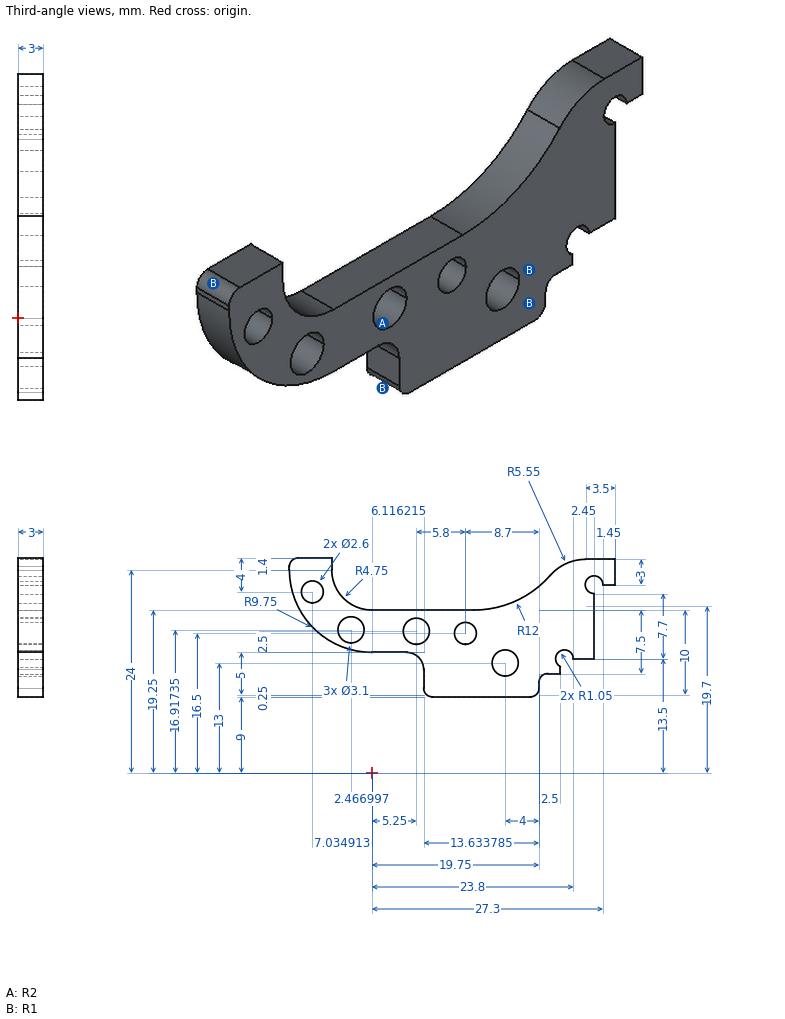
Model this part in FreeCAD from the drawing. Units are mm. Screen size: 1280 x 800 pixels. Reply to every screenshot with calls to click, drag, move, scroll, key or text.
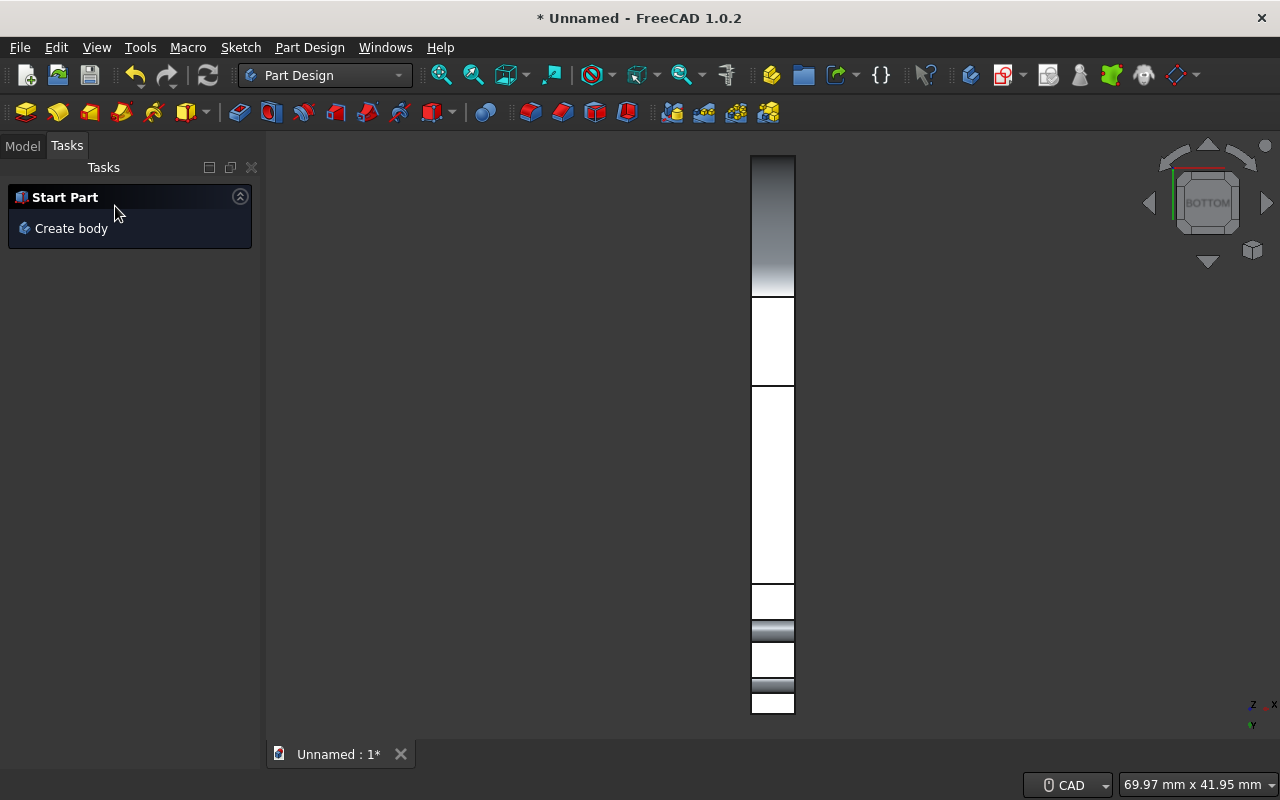
key(4)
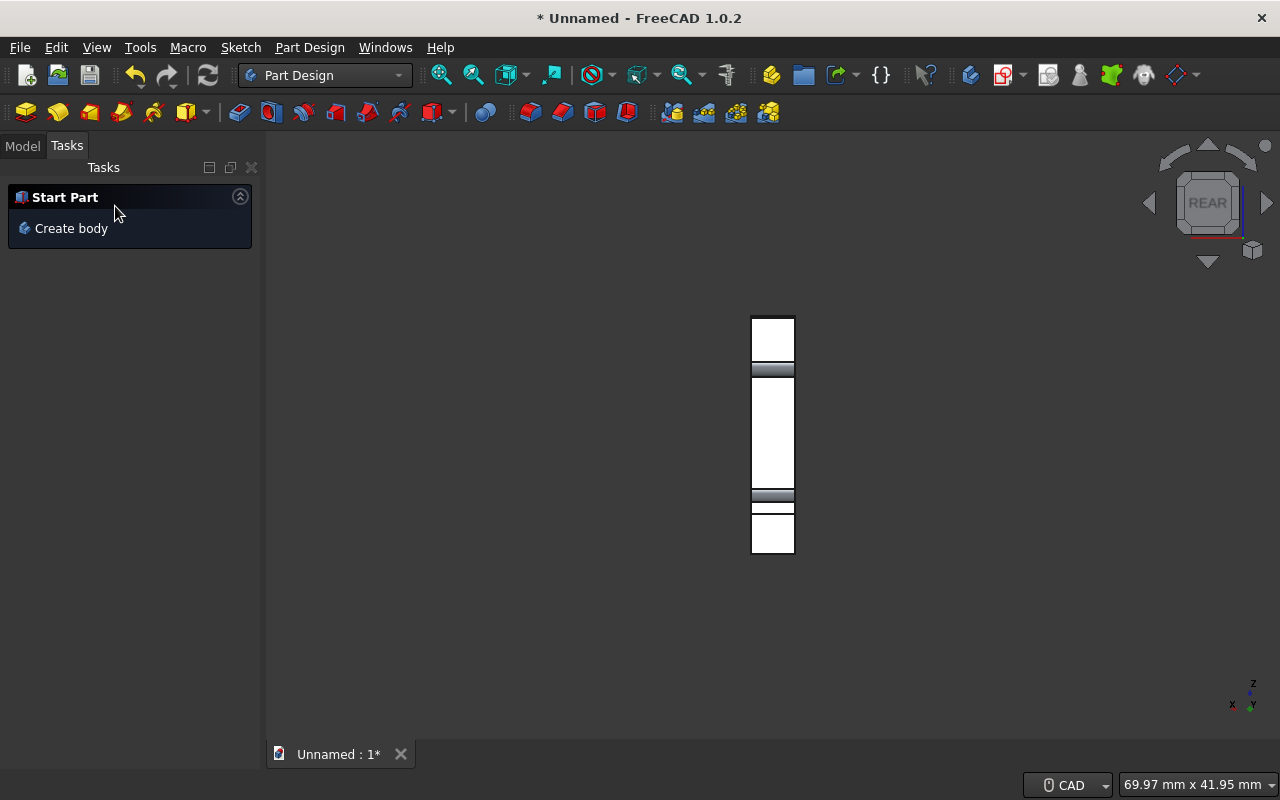
key(v)
key(f)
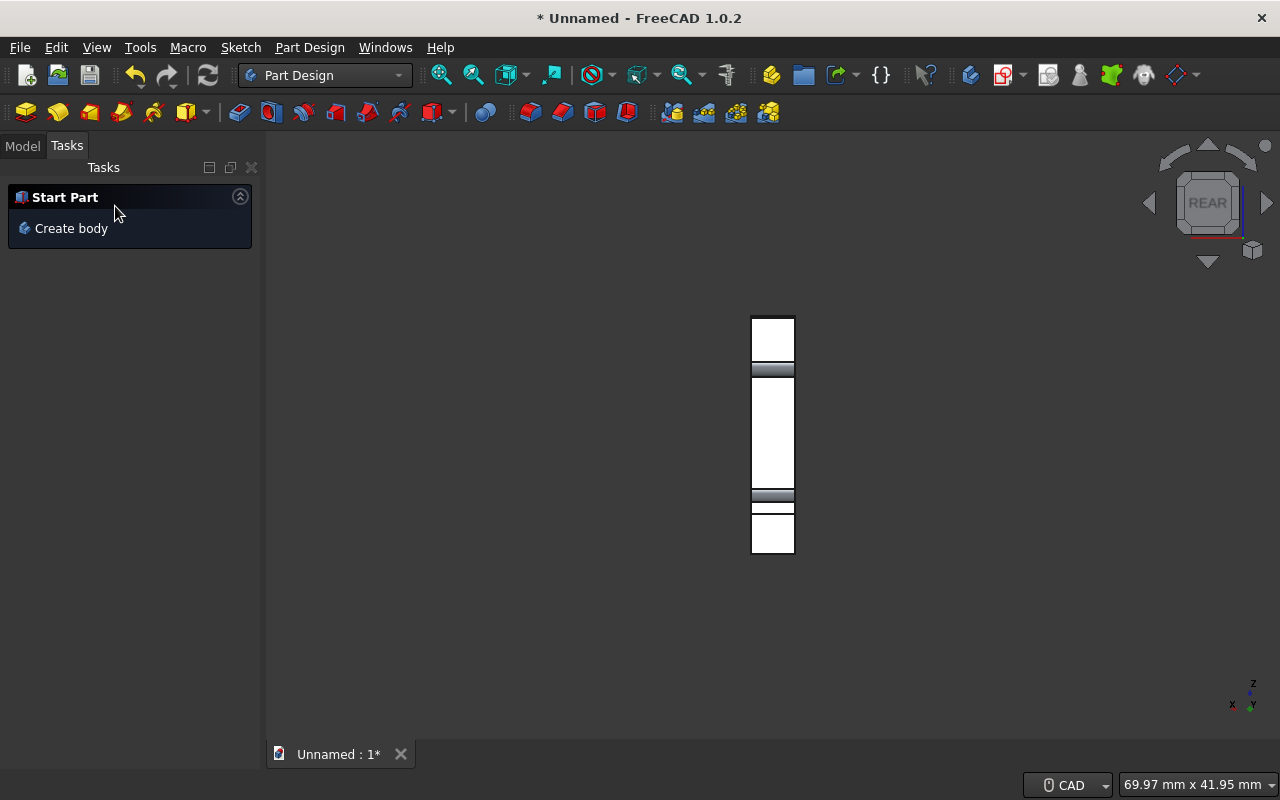
key(6)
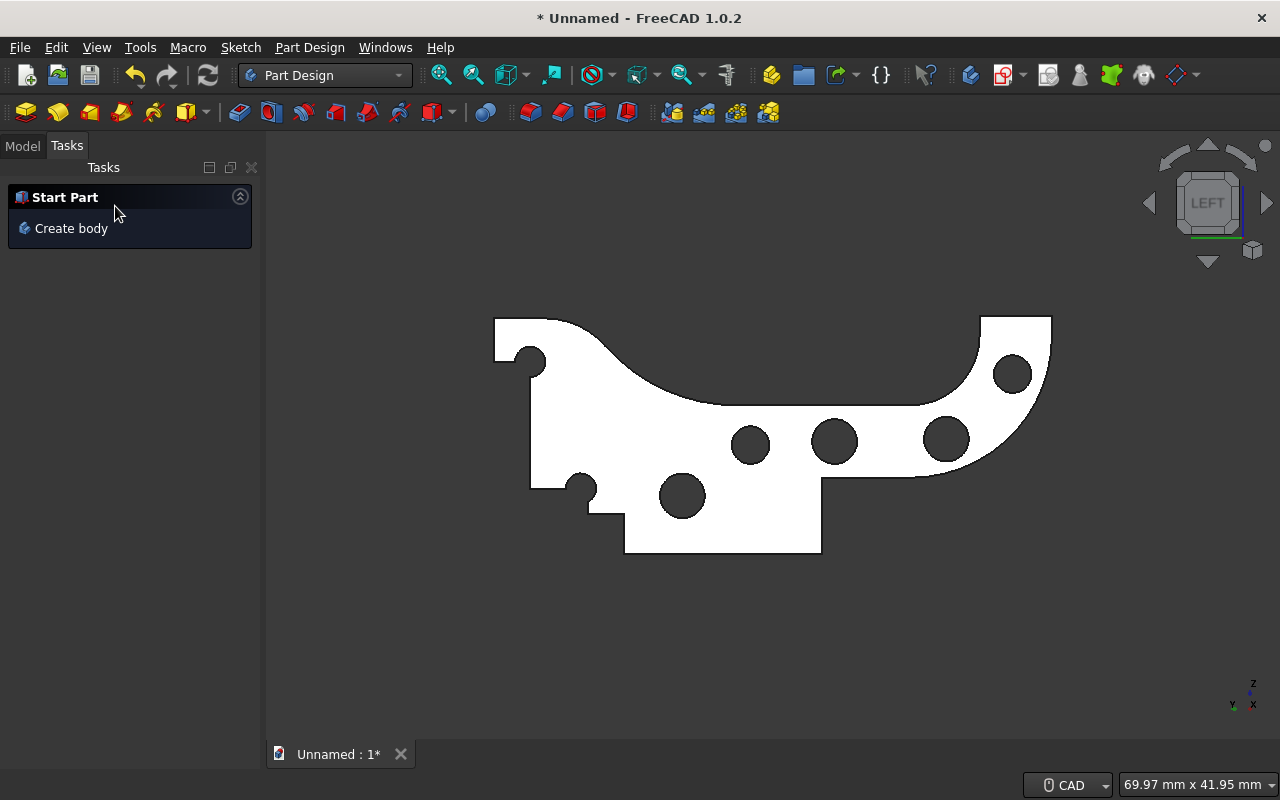
key(v)
key(3)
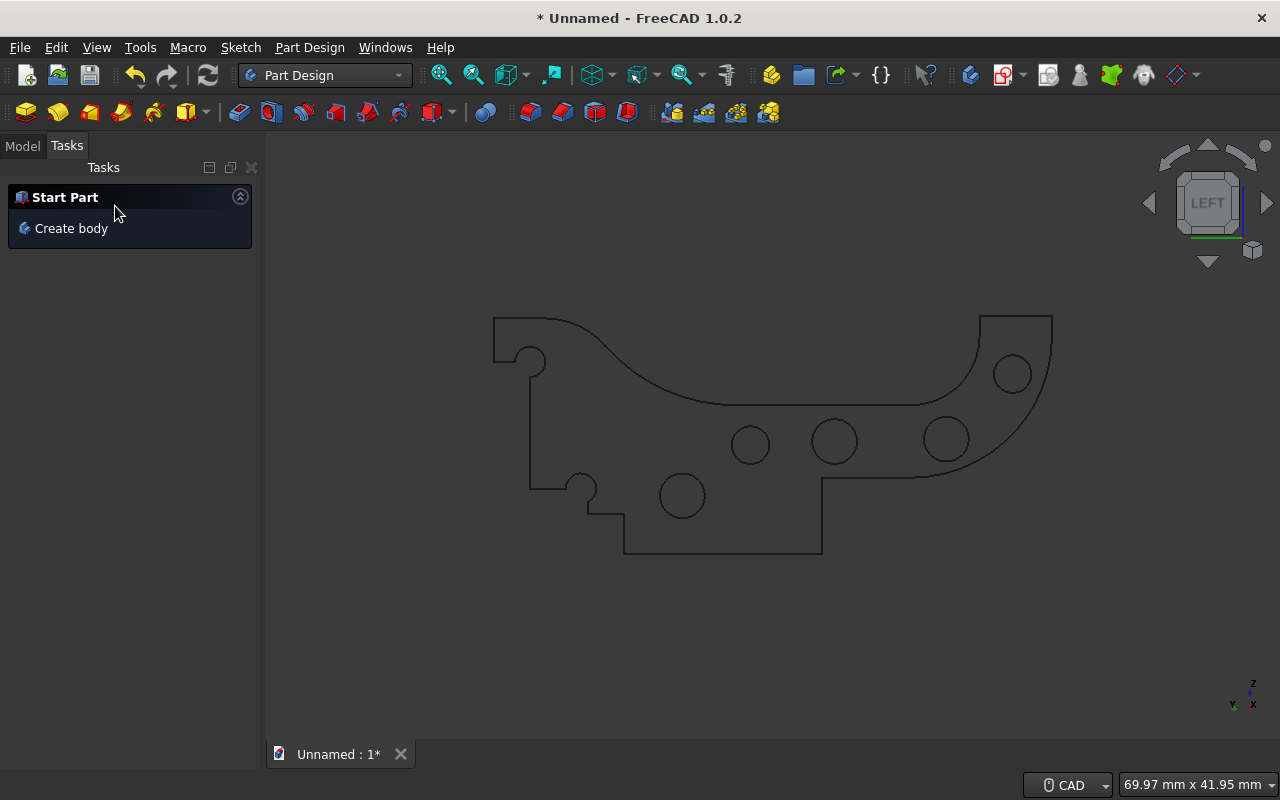
key(0)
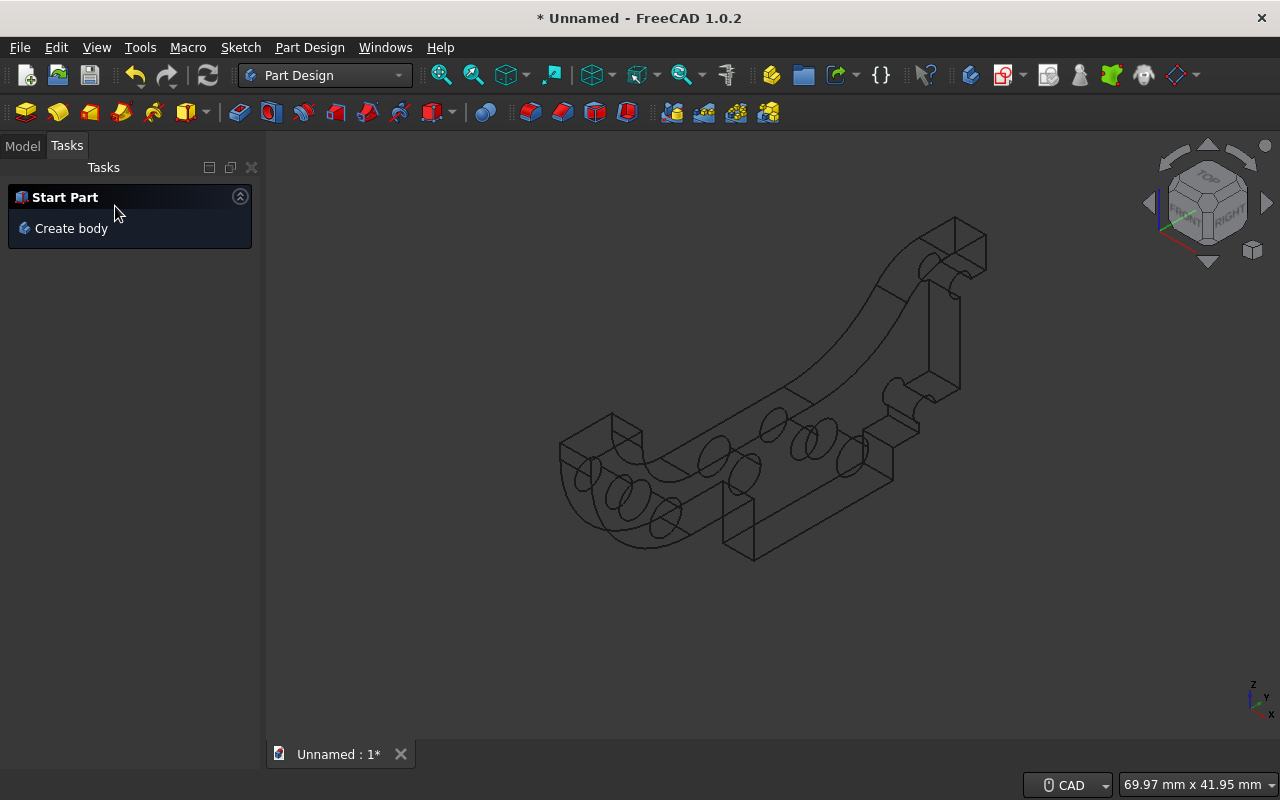
scroll(738, 489, up, 6)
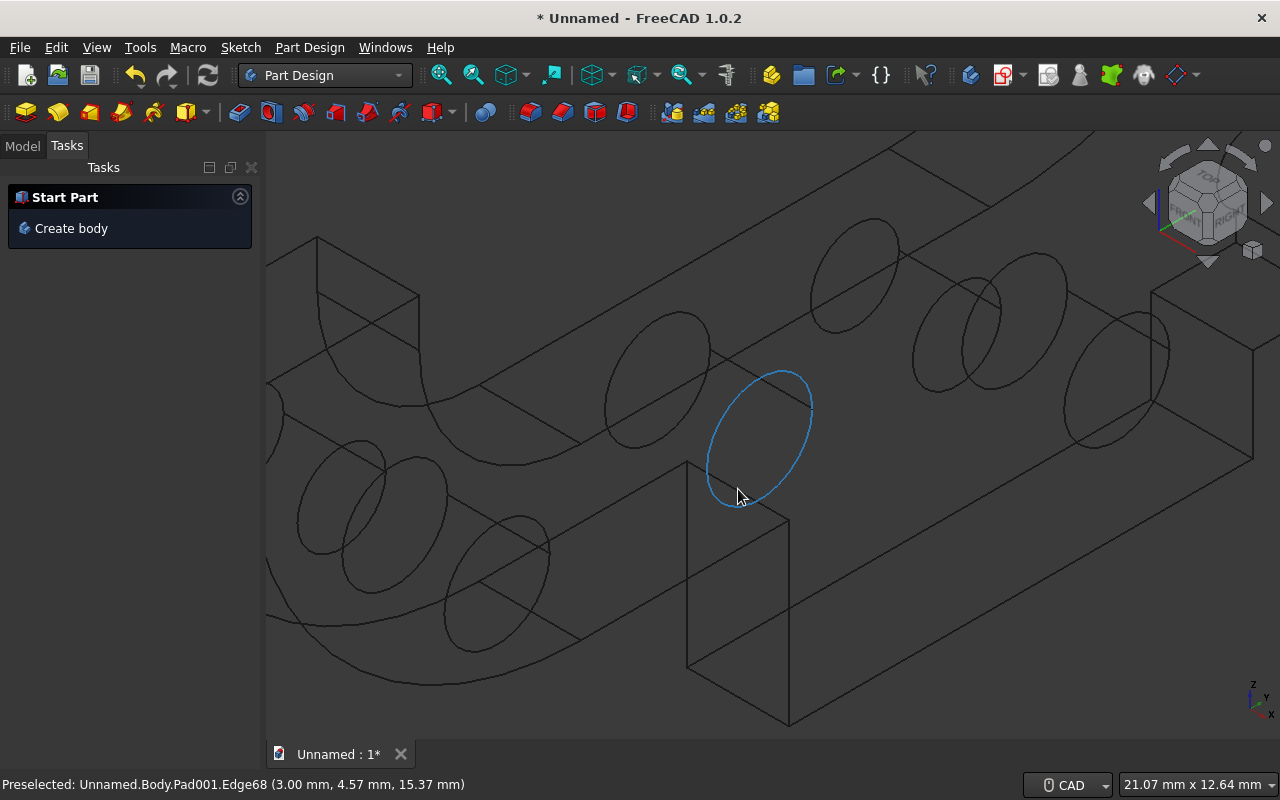
click(738, 490)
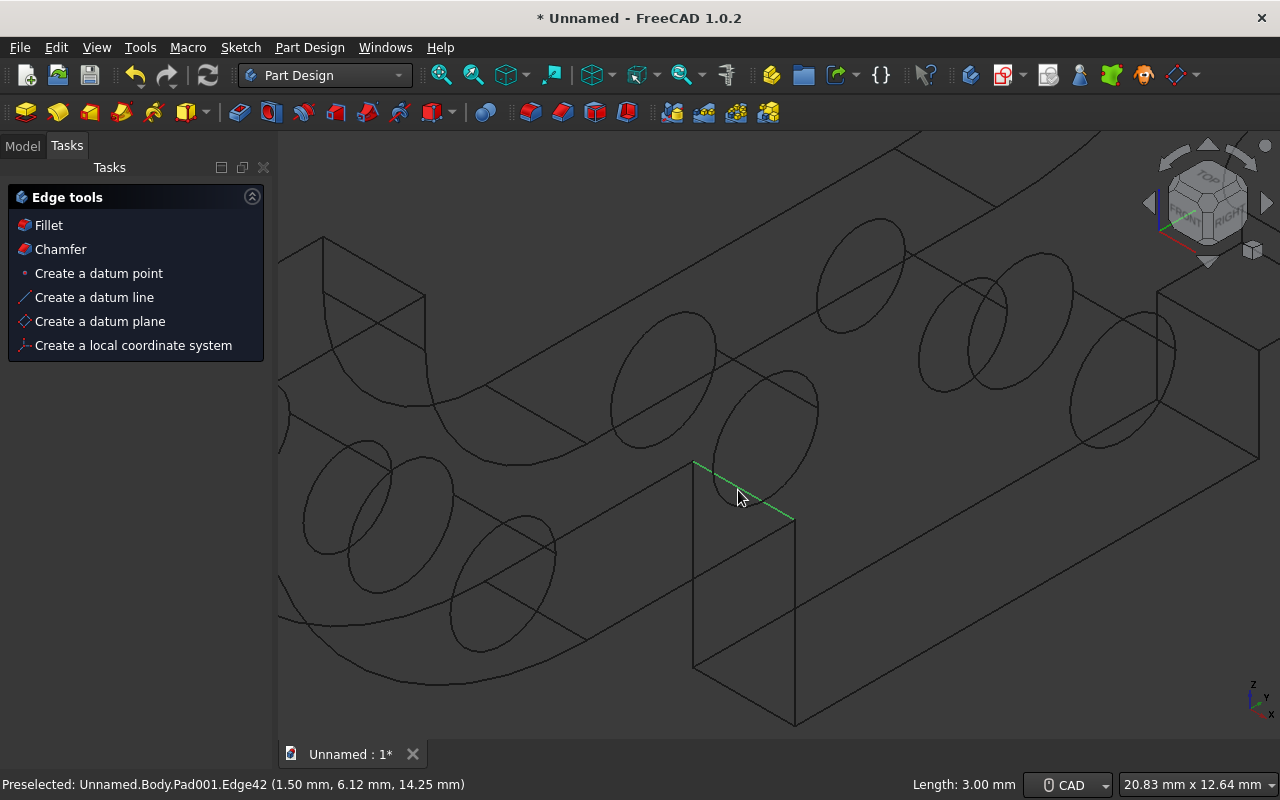
key(v)
key(1)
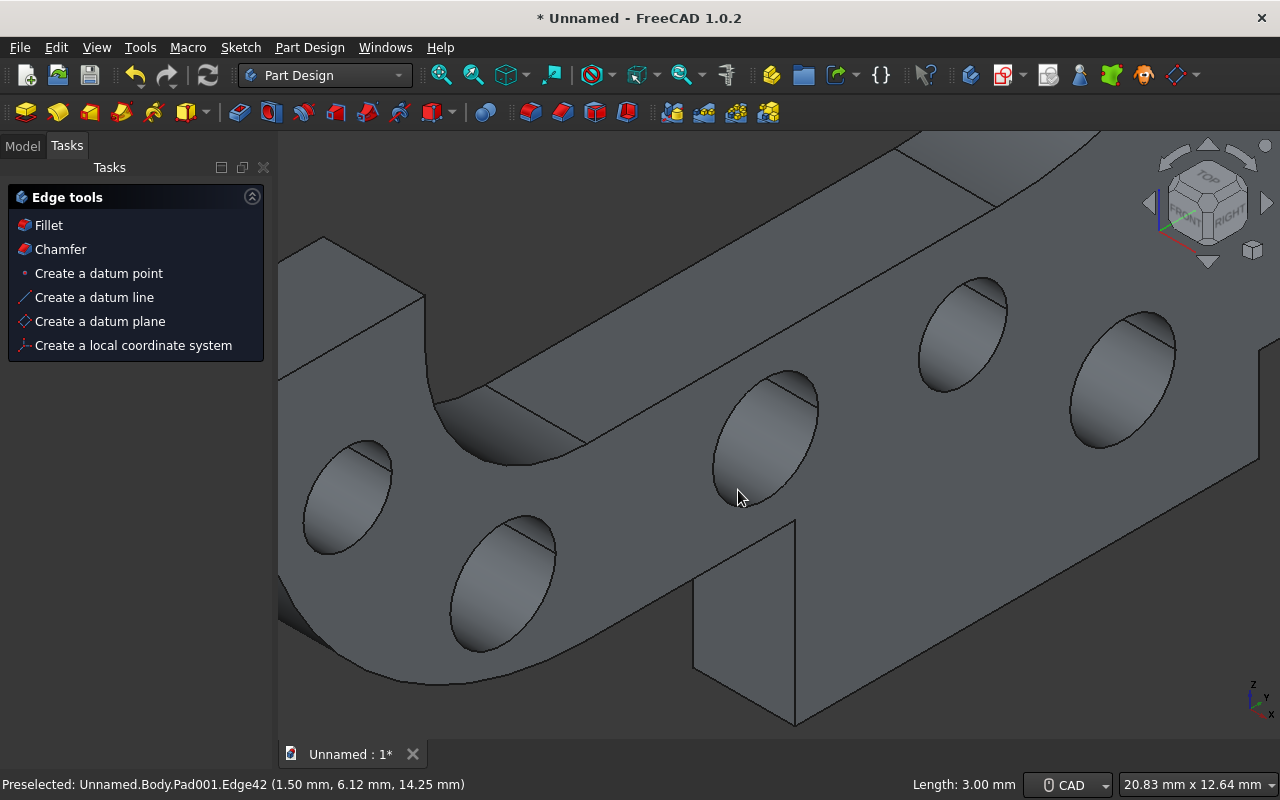
click(532, 112)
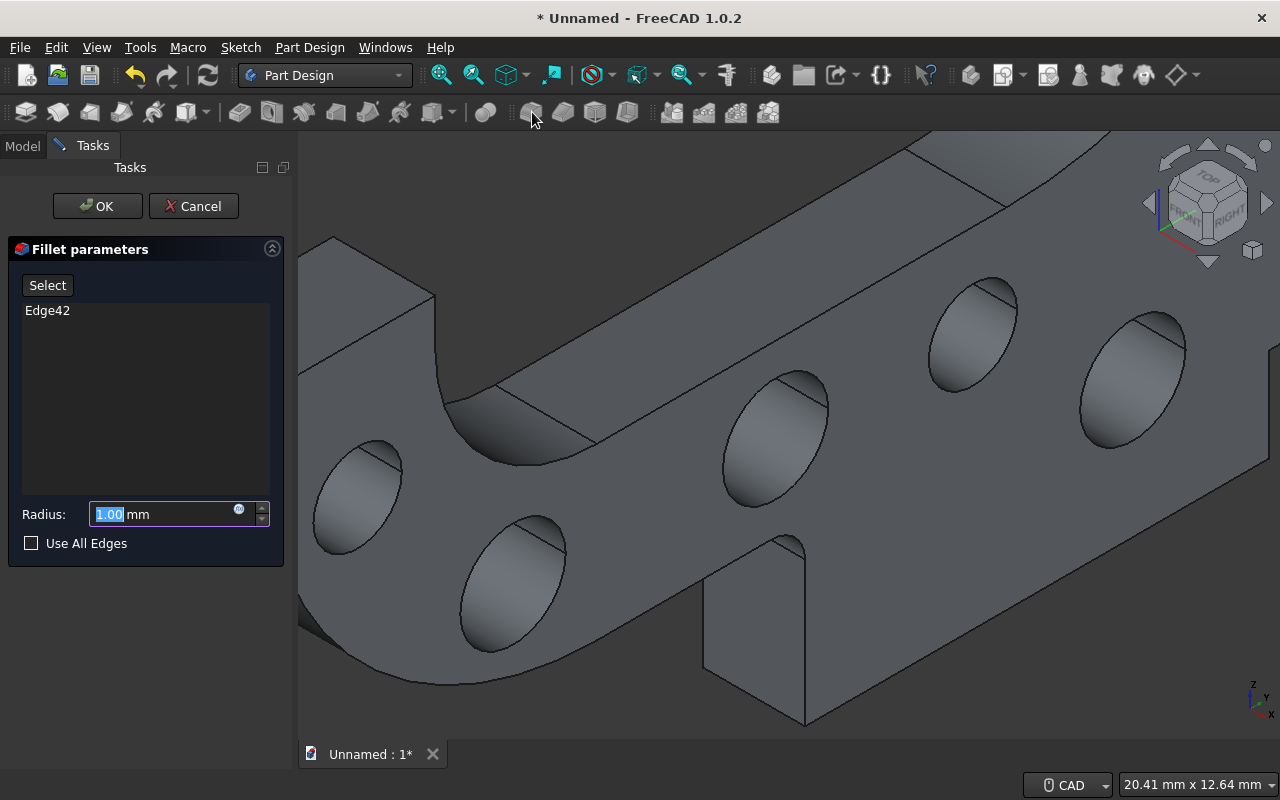
text(2)
key(Tab)